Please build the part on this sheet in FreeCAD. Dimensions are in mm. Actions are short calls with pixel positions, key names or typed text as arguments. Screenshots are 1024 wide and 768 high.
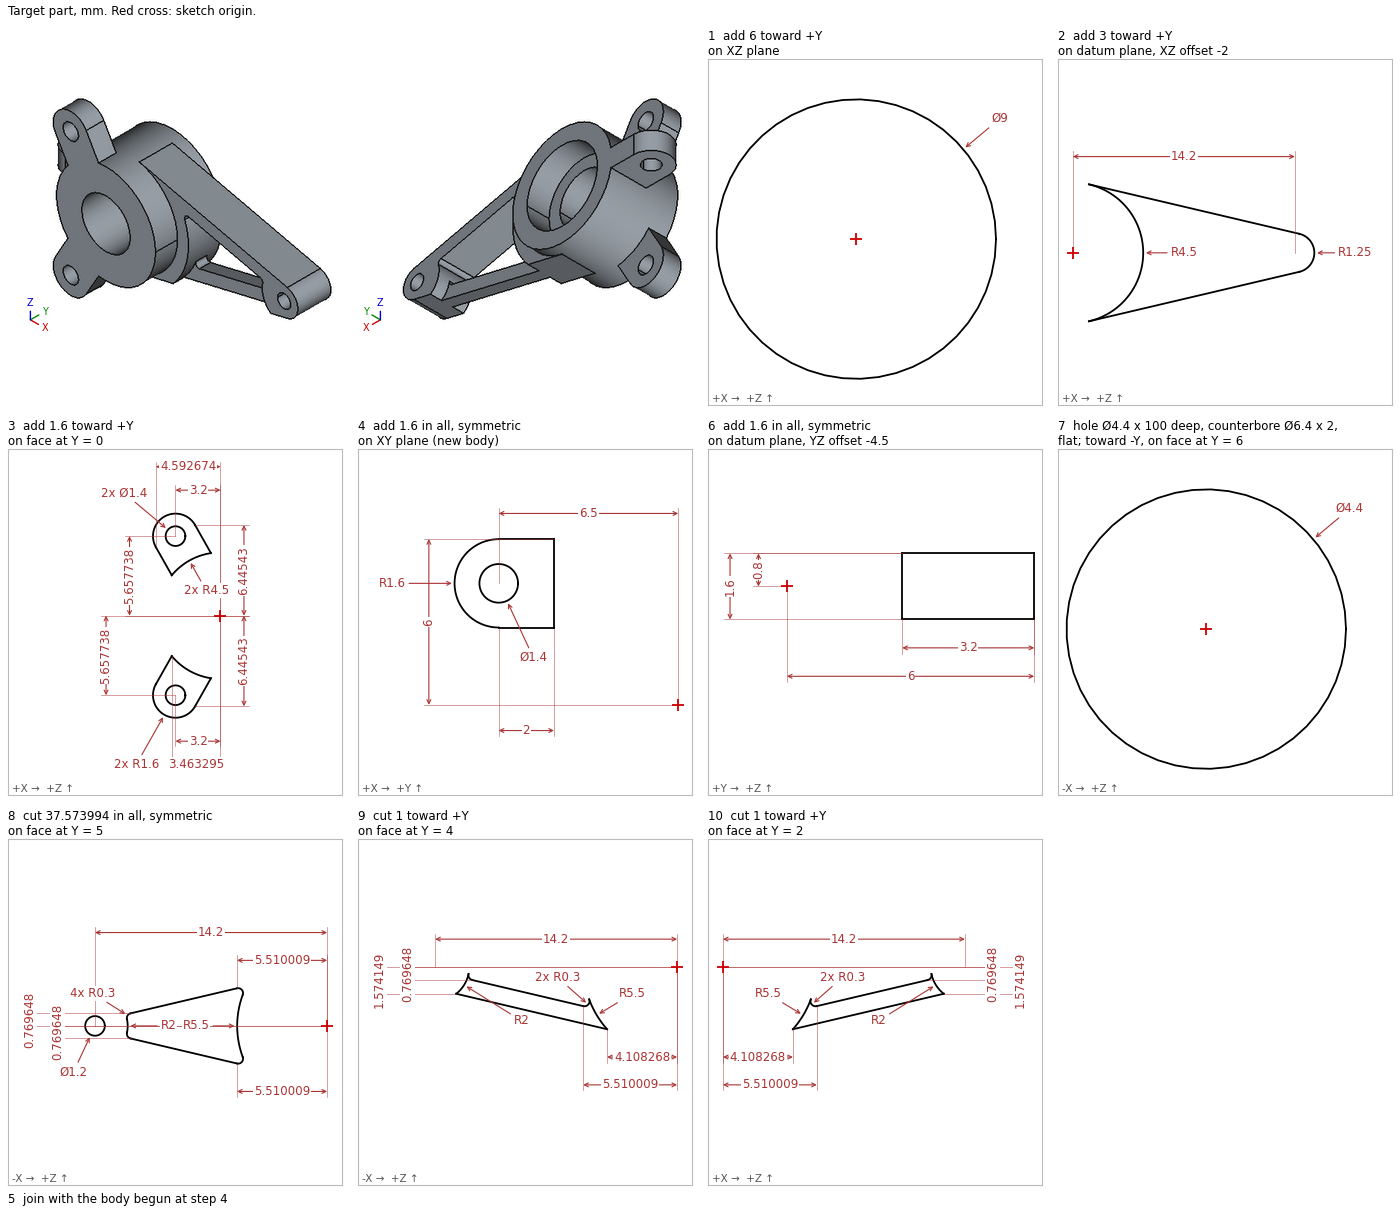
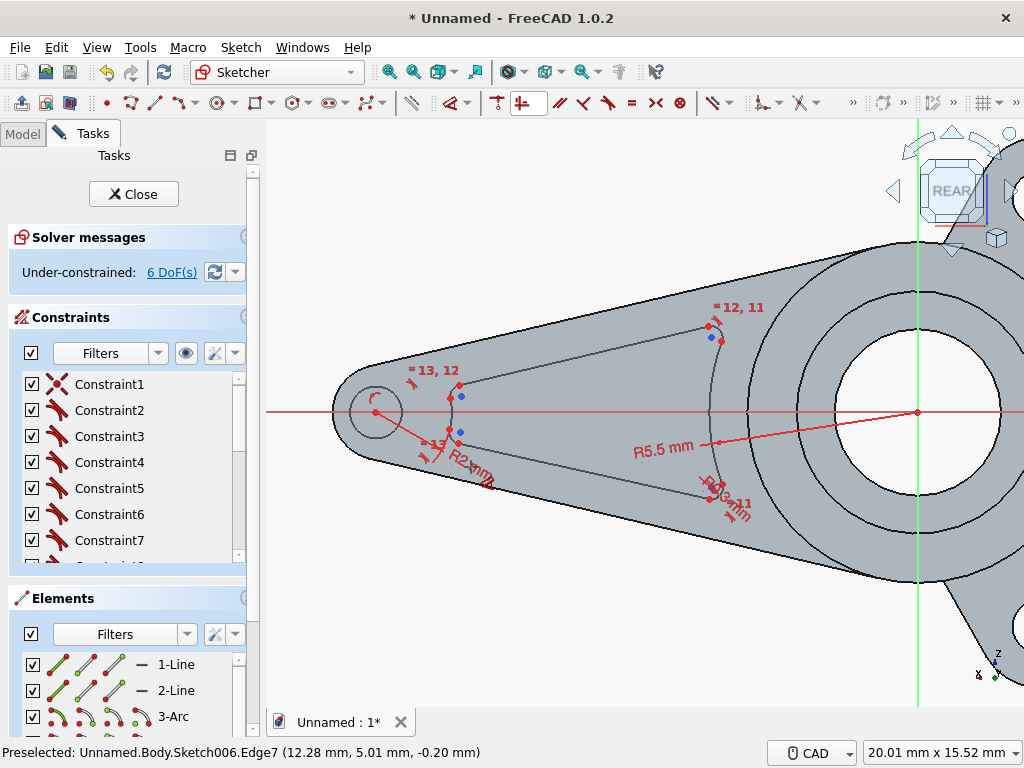
click(394, 394)
click(416, 371)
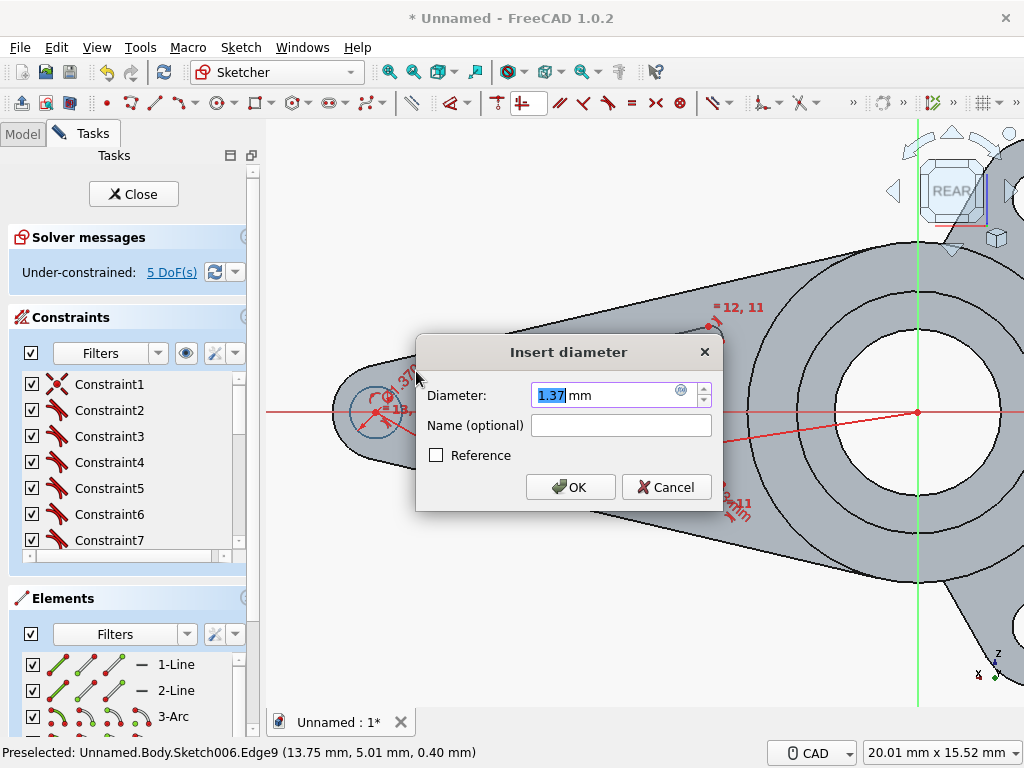
text(1.2)
key(Return)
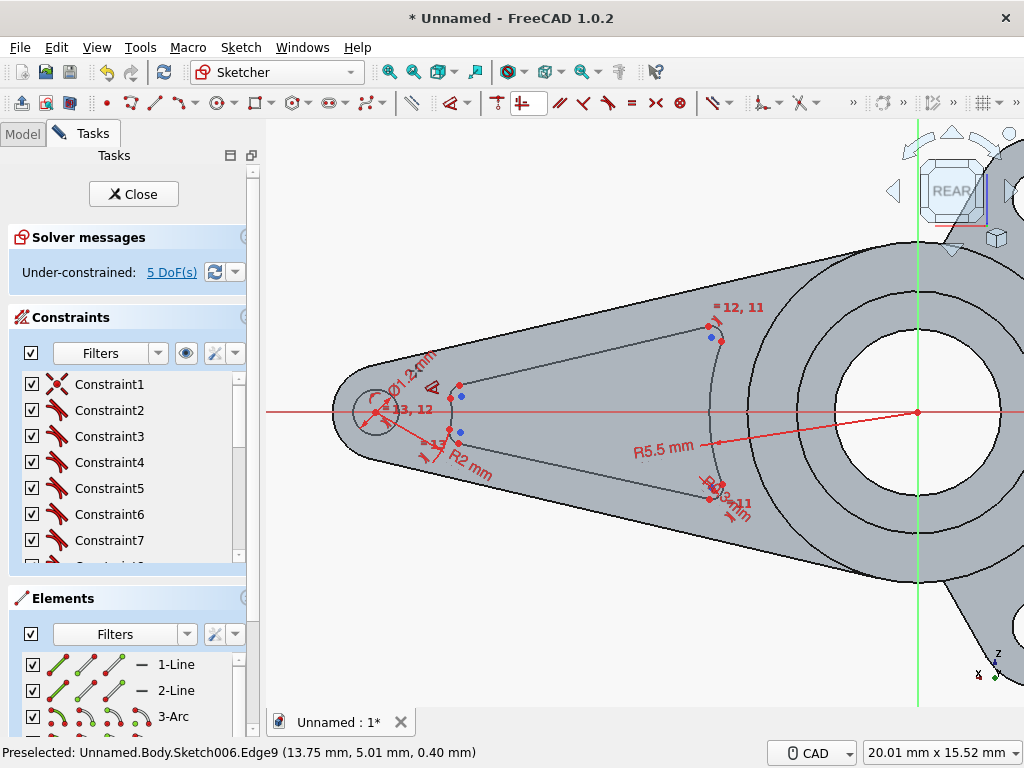
click(376, 412)
click(787, 446)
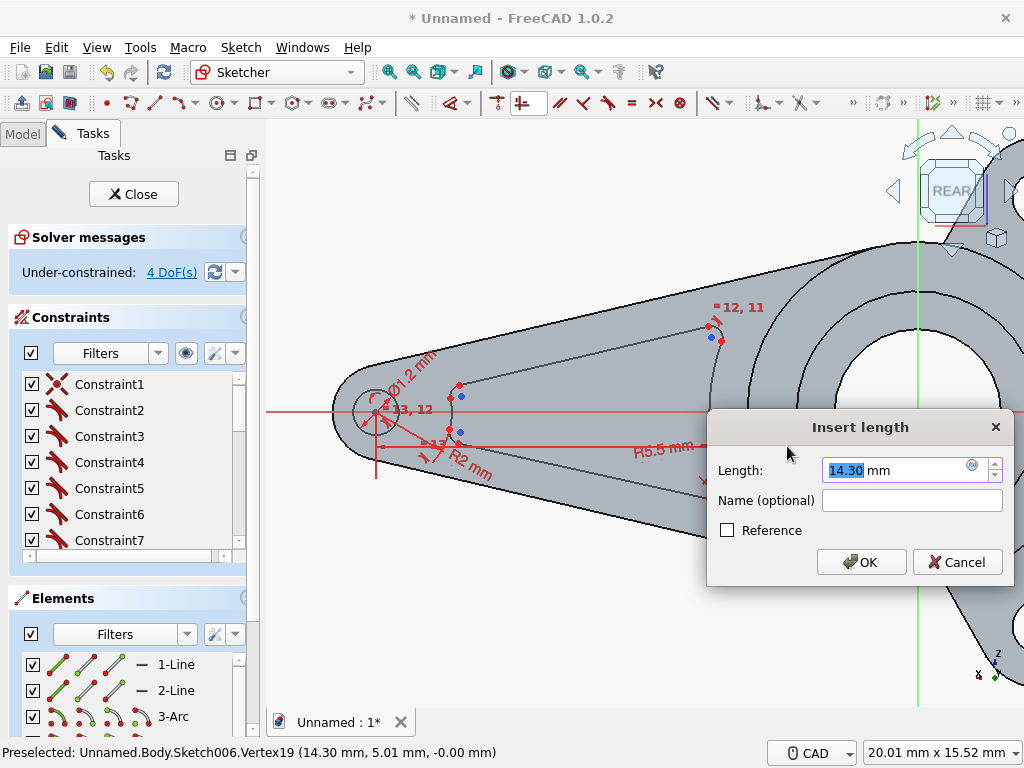
text(14.2)
key(Return)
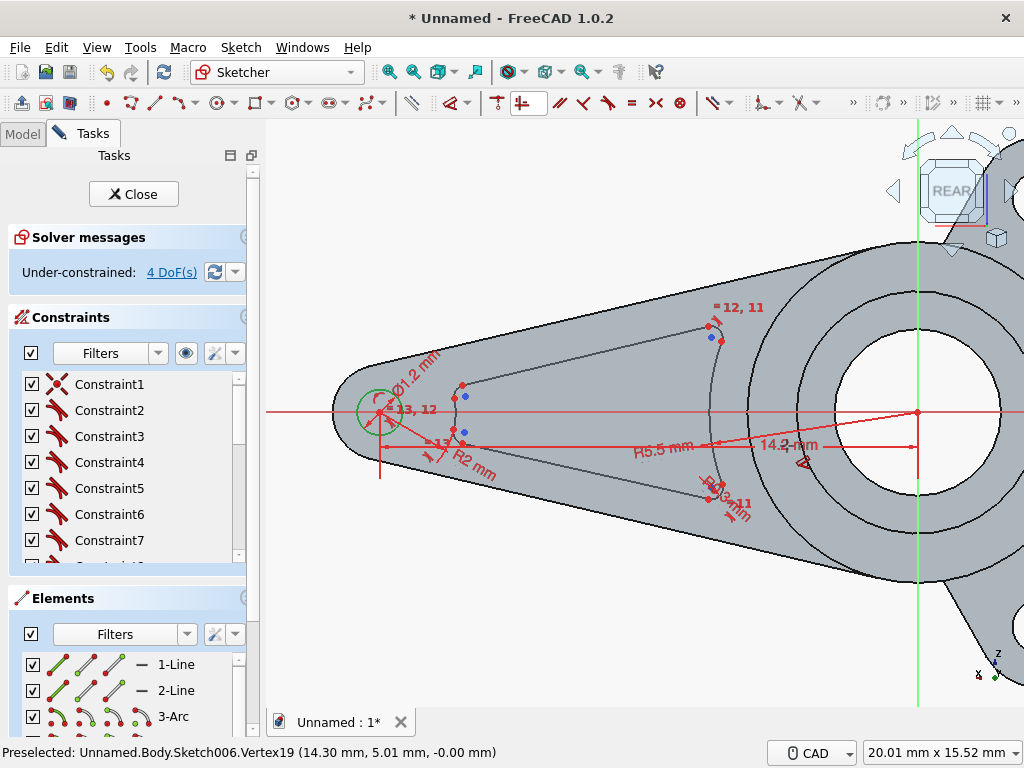
scroll(462, 444, up, 2)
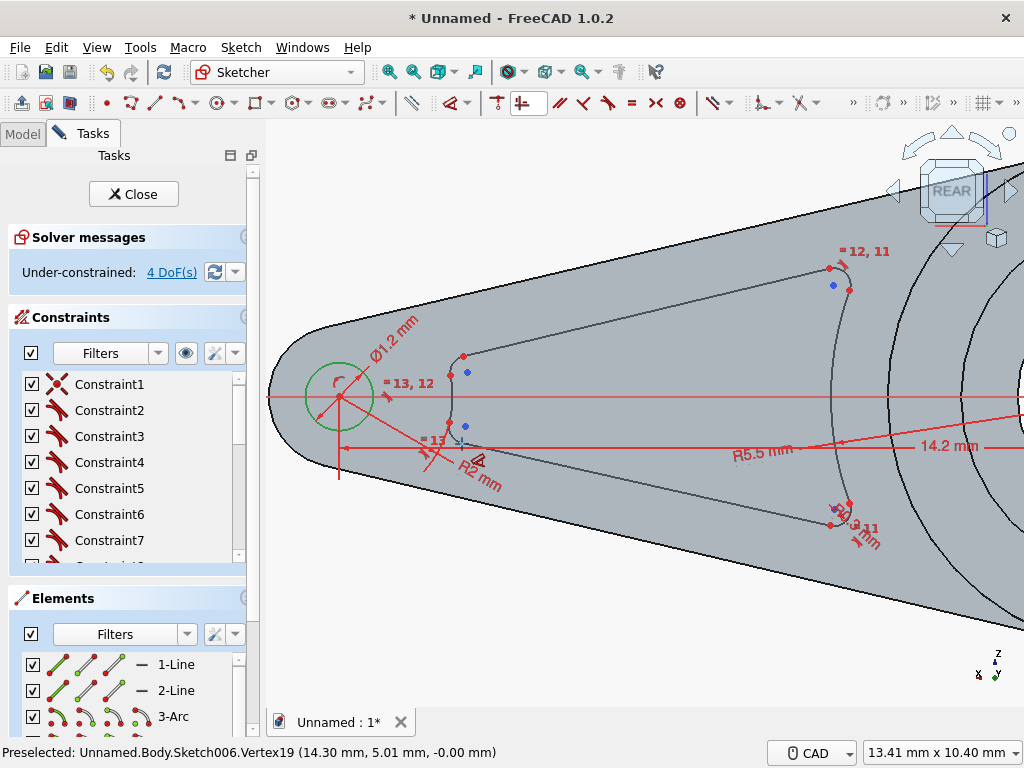
click(462, 443)
click(428, 420)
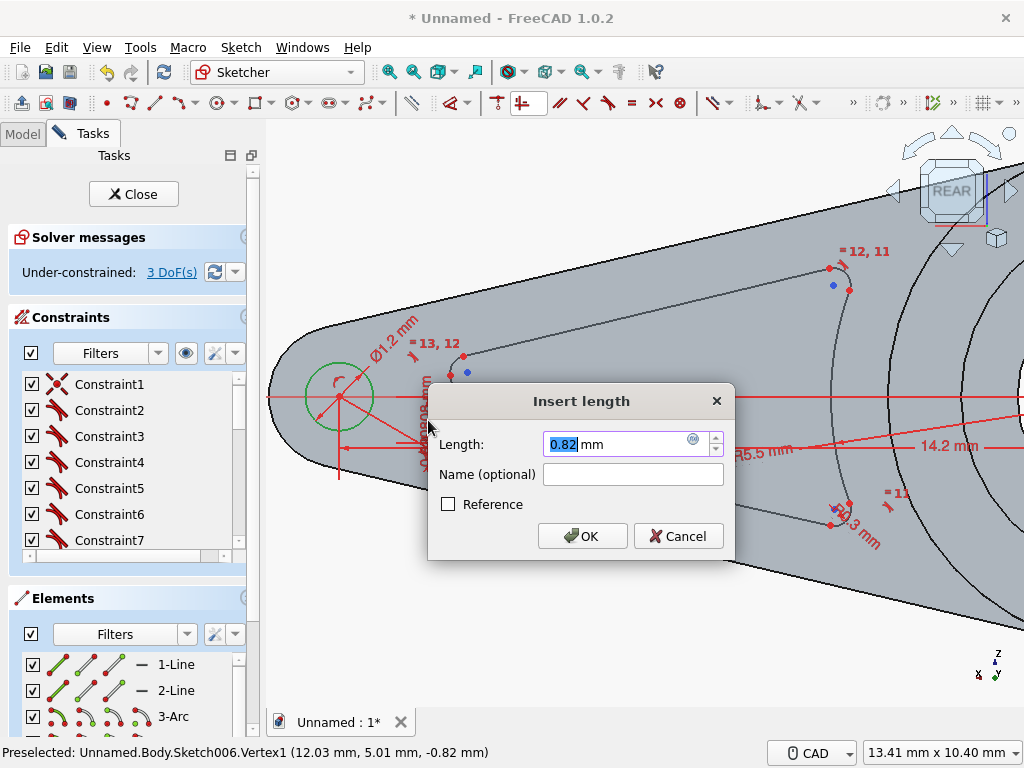
text(0.769648)
key(Return)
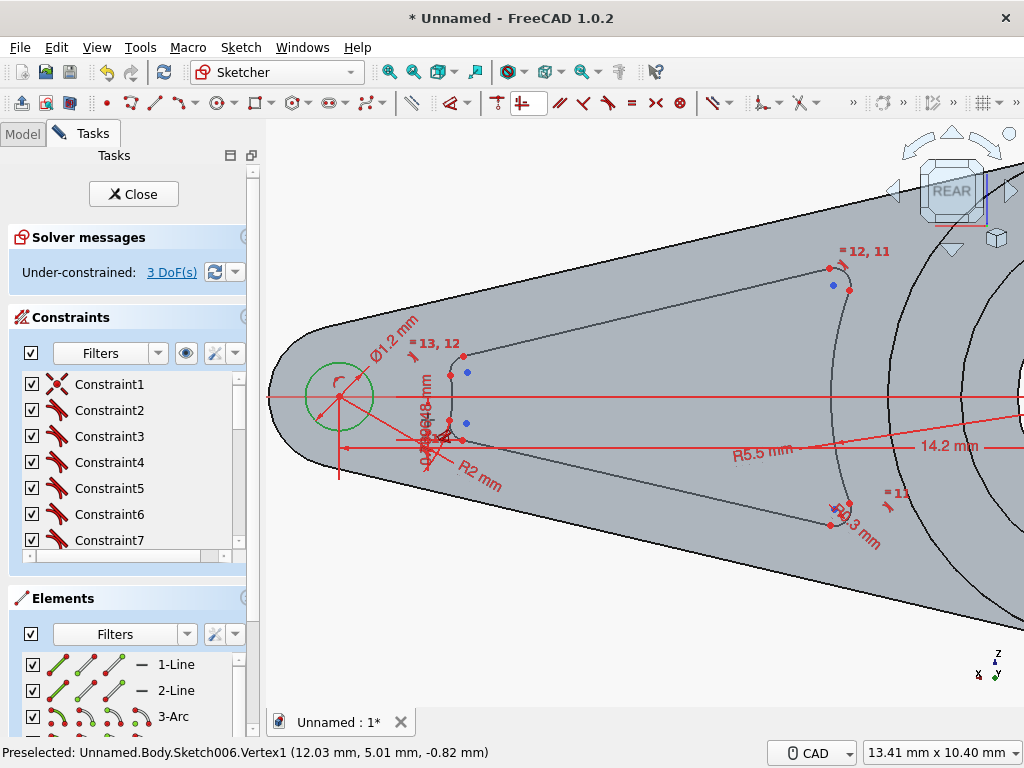
click(830, 526)
click(845, 560)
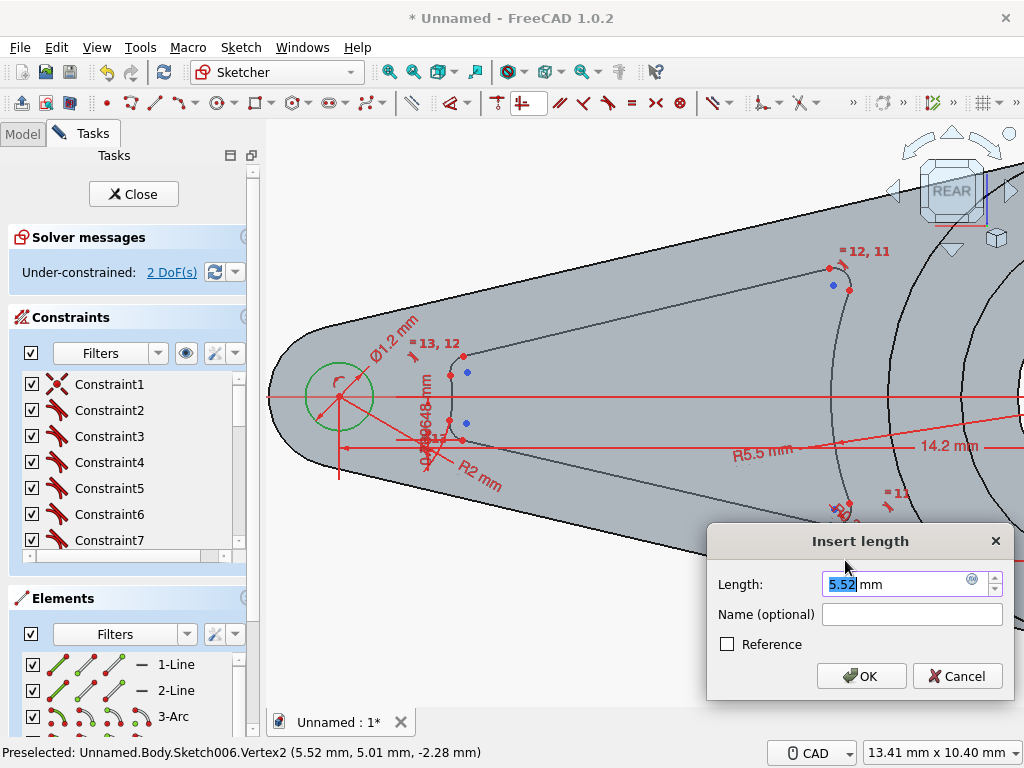
text(5.510009)
key(Return)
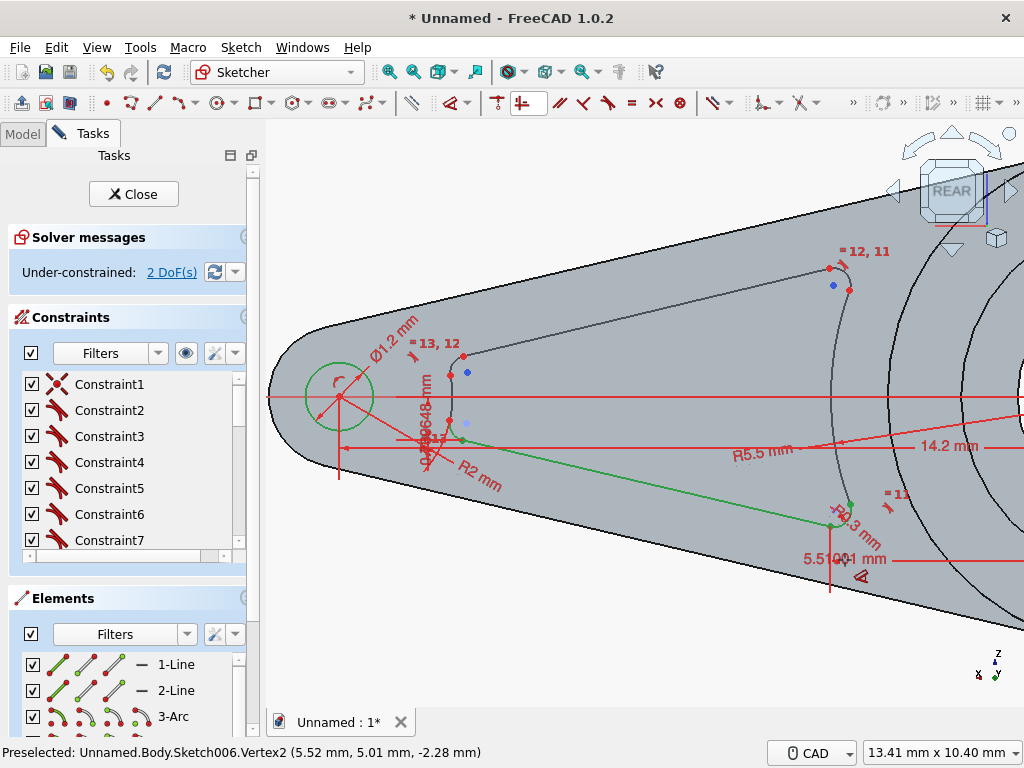
click(830, 269)
click(844, 235)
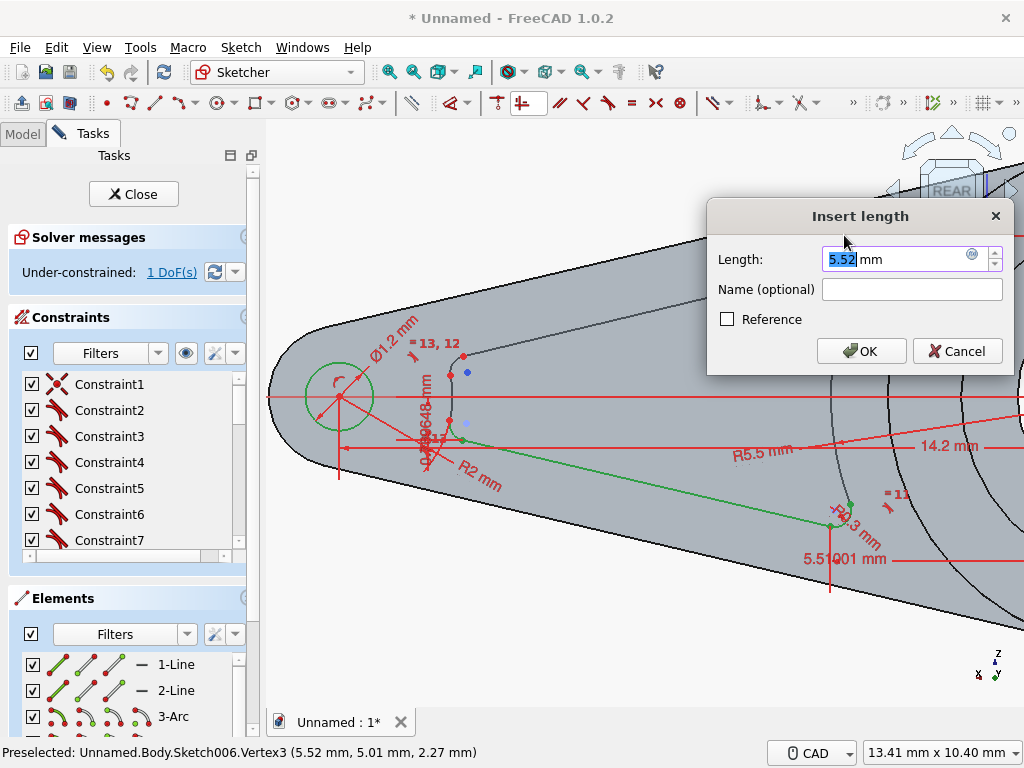
text(5.510009)
key(Return)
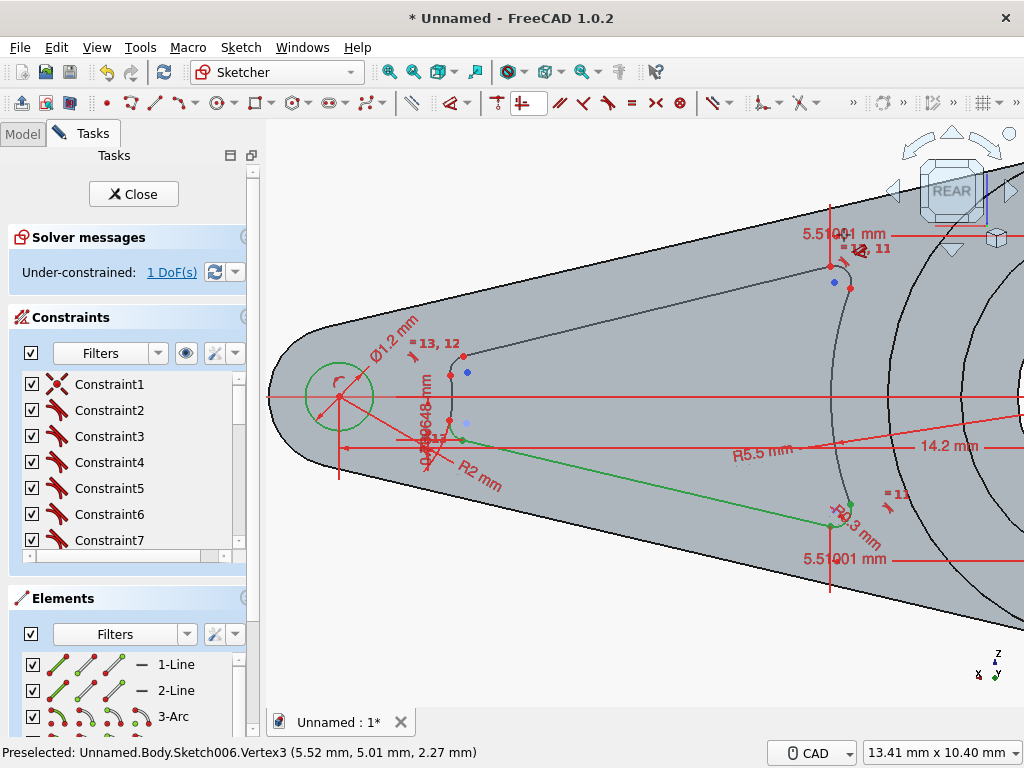
click(463, 356)
click(429, 377)